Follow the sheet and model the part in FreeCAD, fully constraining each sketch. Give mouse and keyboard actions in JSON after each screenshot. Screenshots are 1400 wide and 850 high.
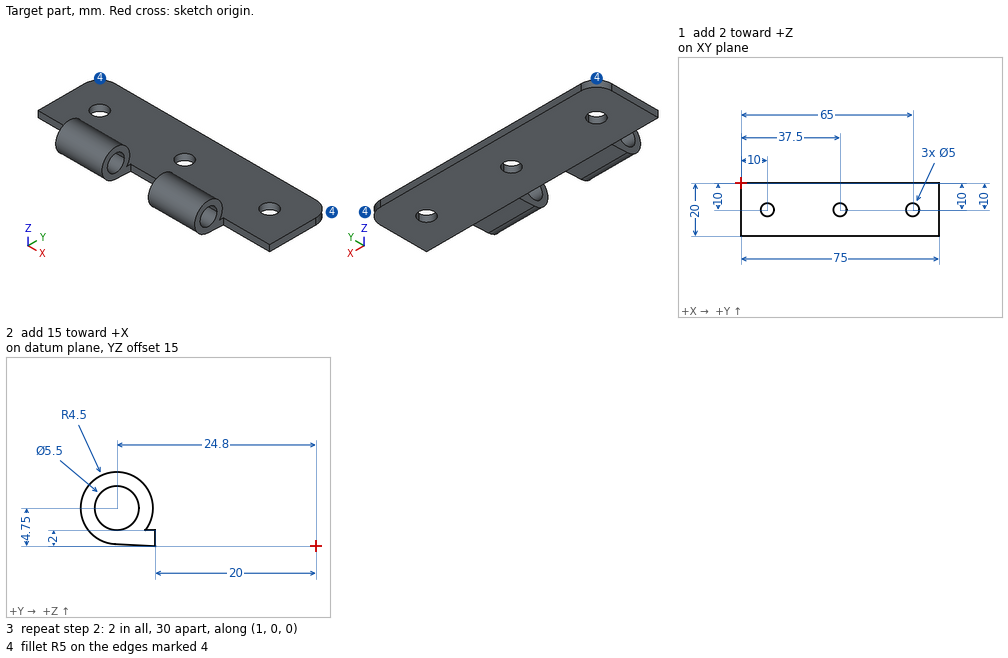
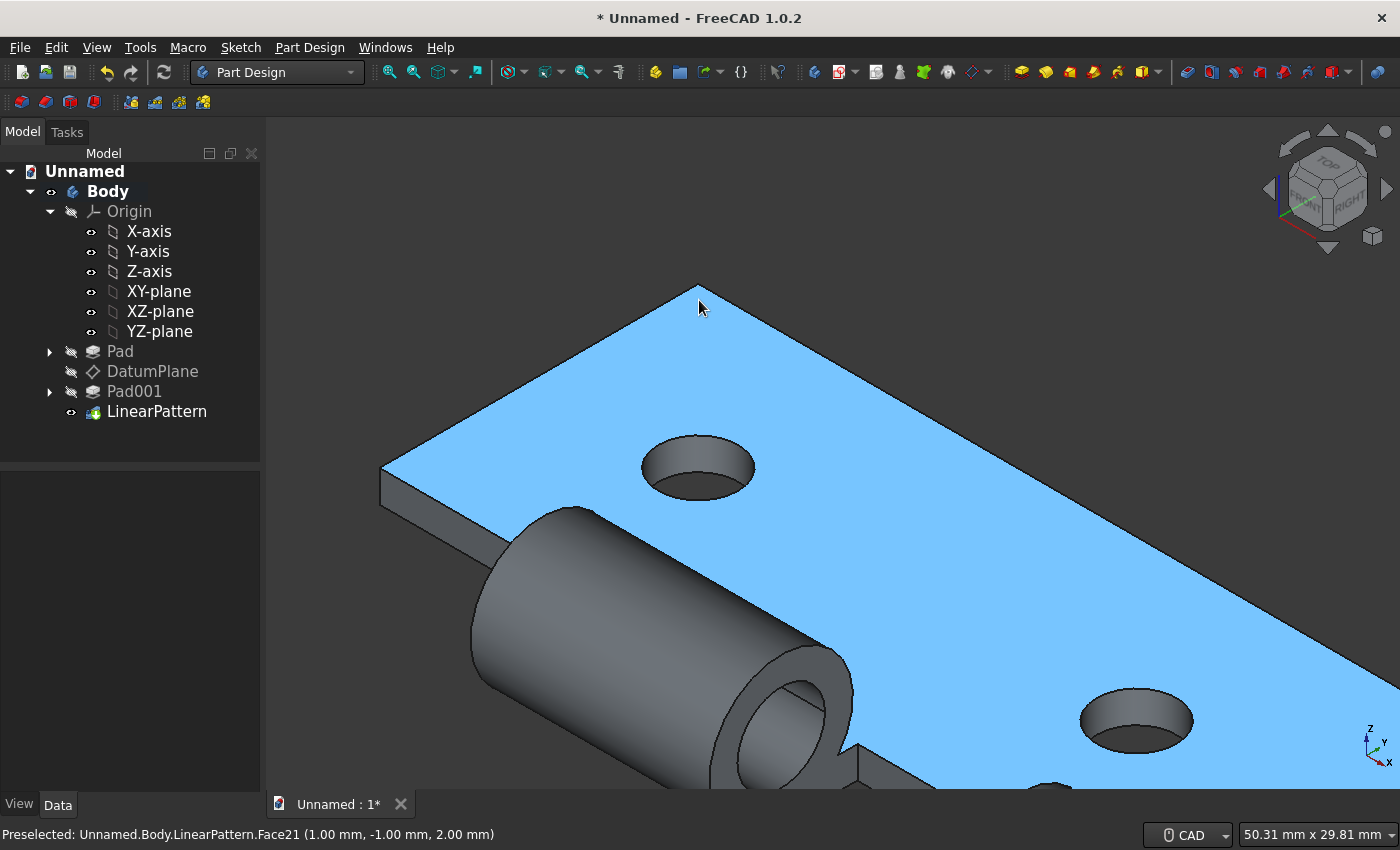
{"action": "key", "text": "v f"}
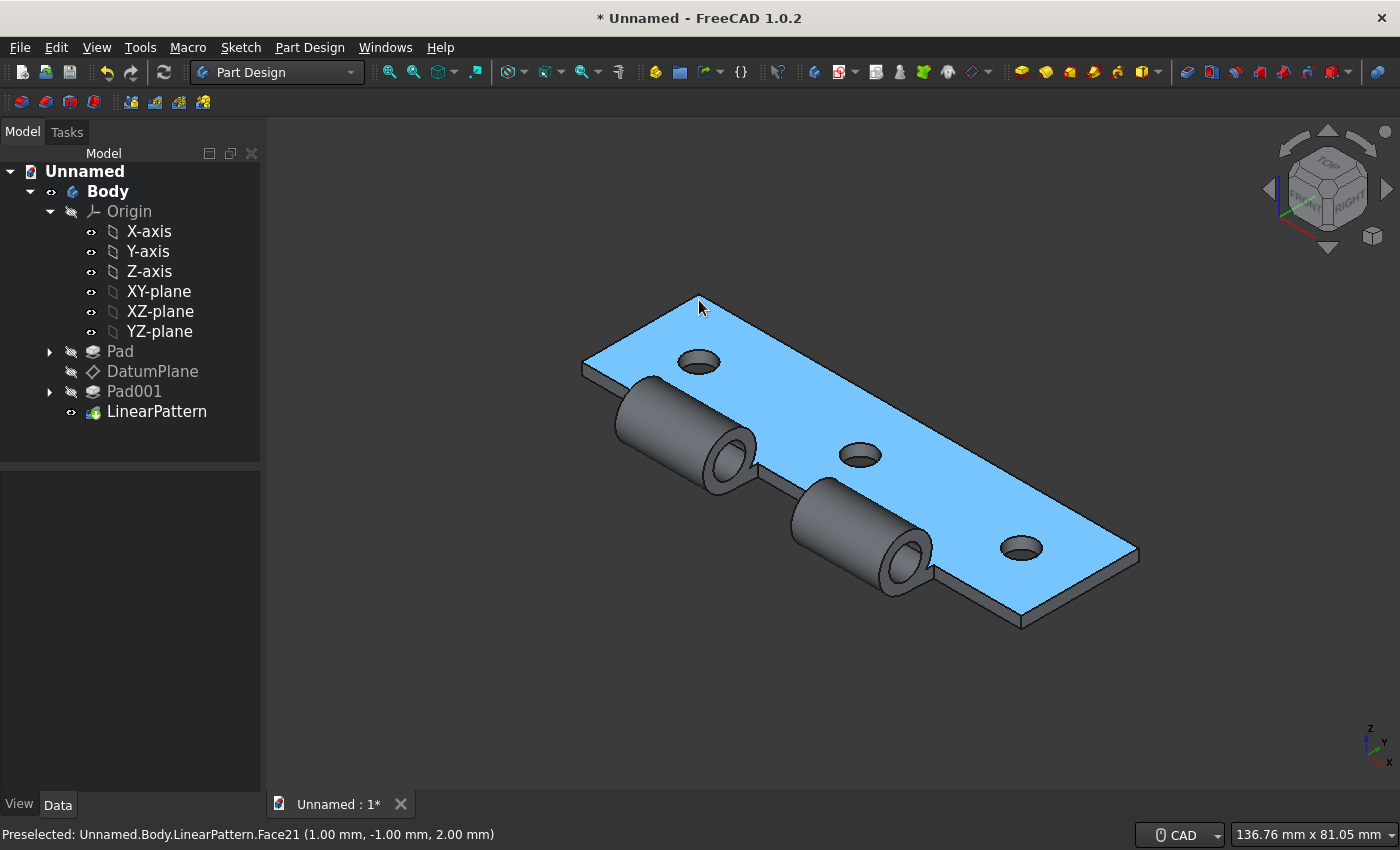
{"action": "key", "text": "2"}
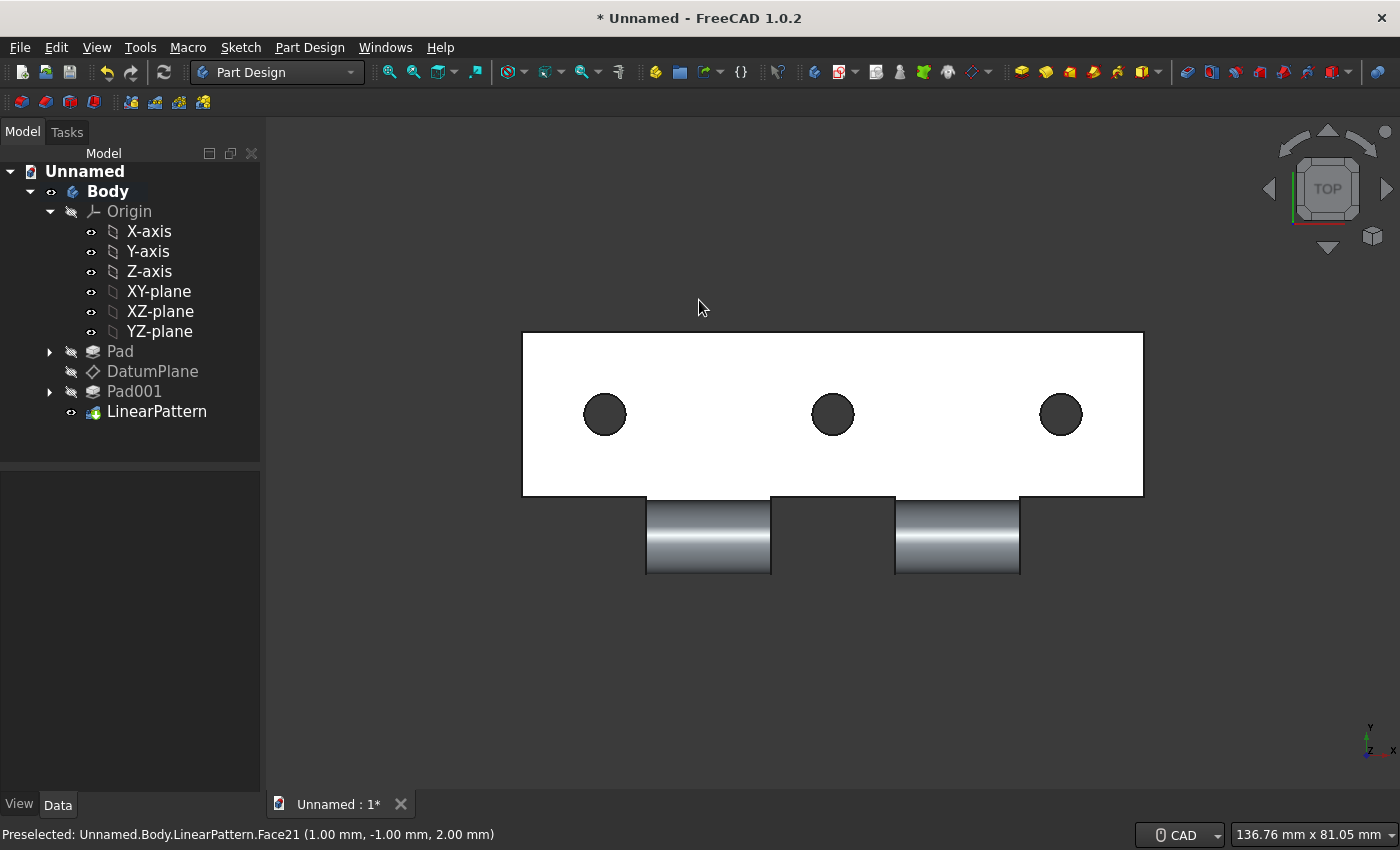
{"action": "scroll", "coordinate": [522, 331], "scroll_direction": "up", "scroll_amount": 5}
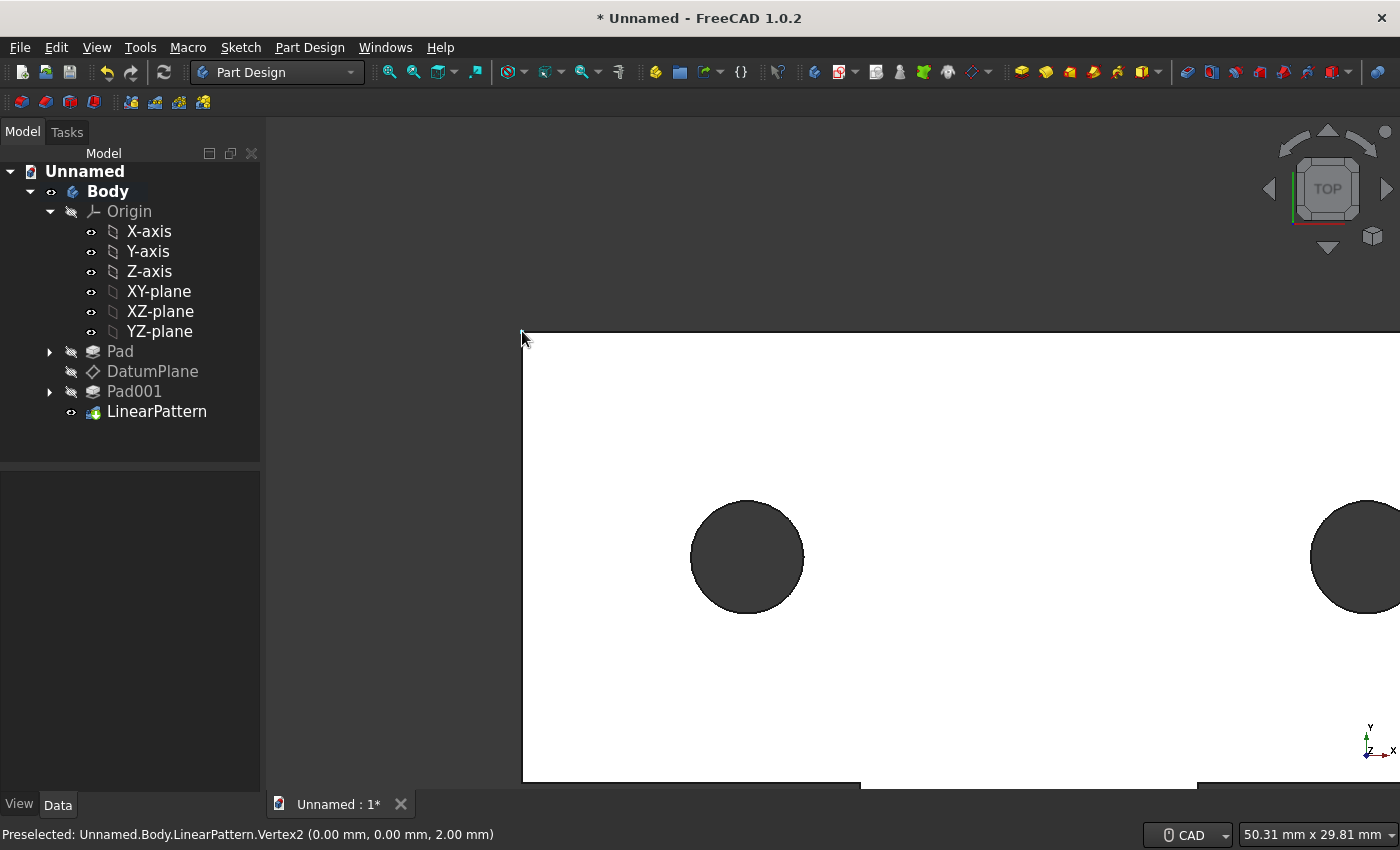
{"action": "key", "text": "v f"}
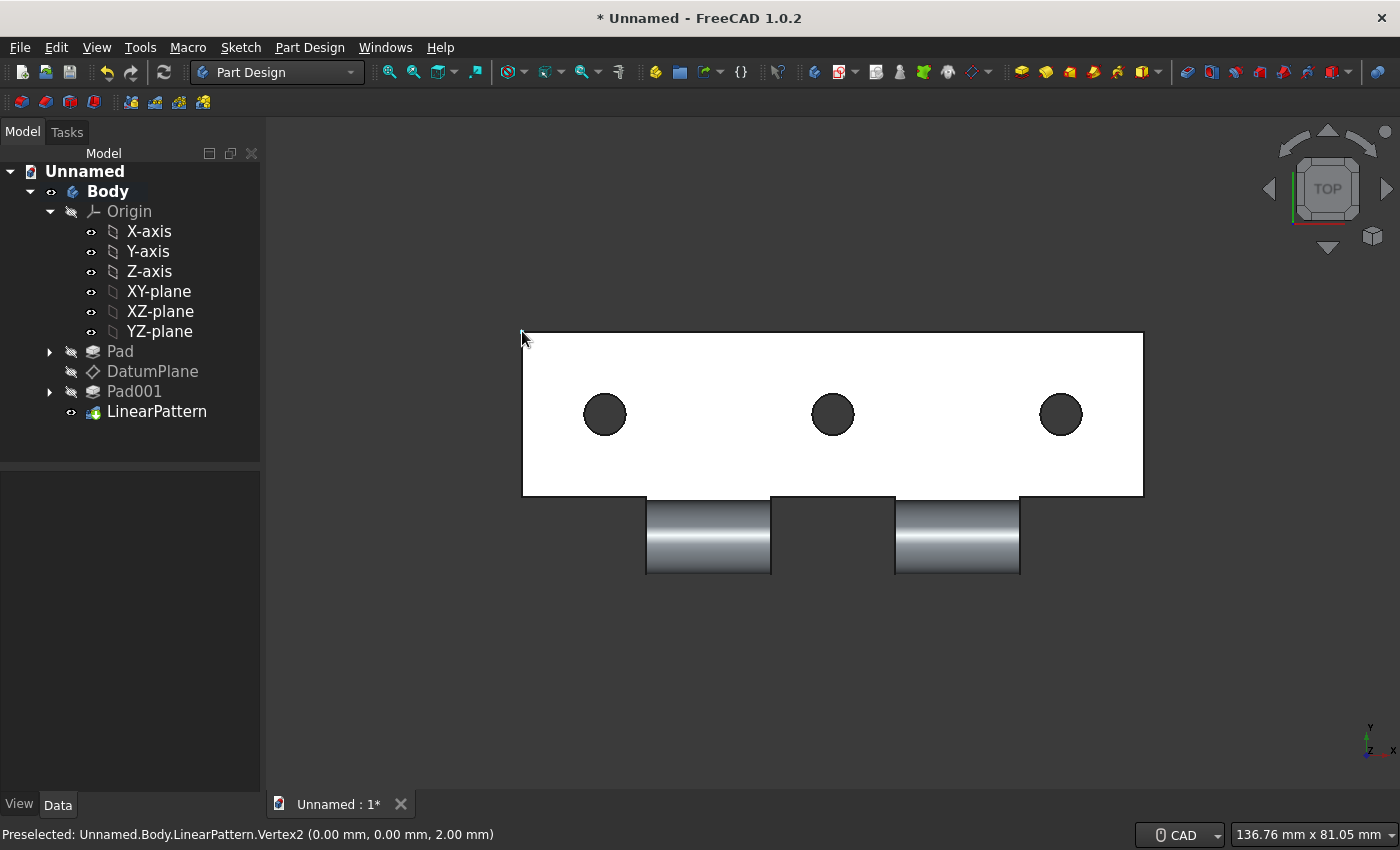
{"action": "key", "text": "1"}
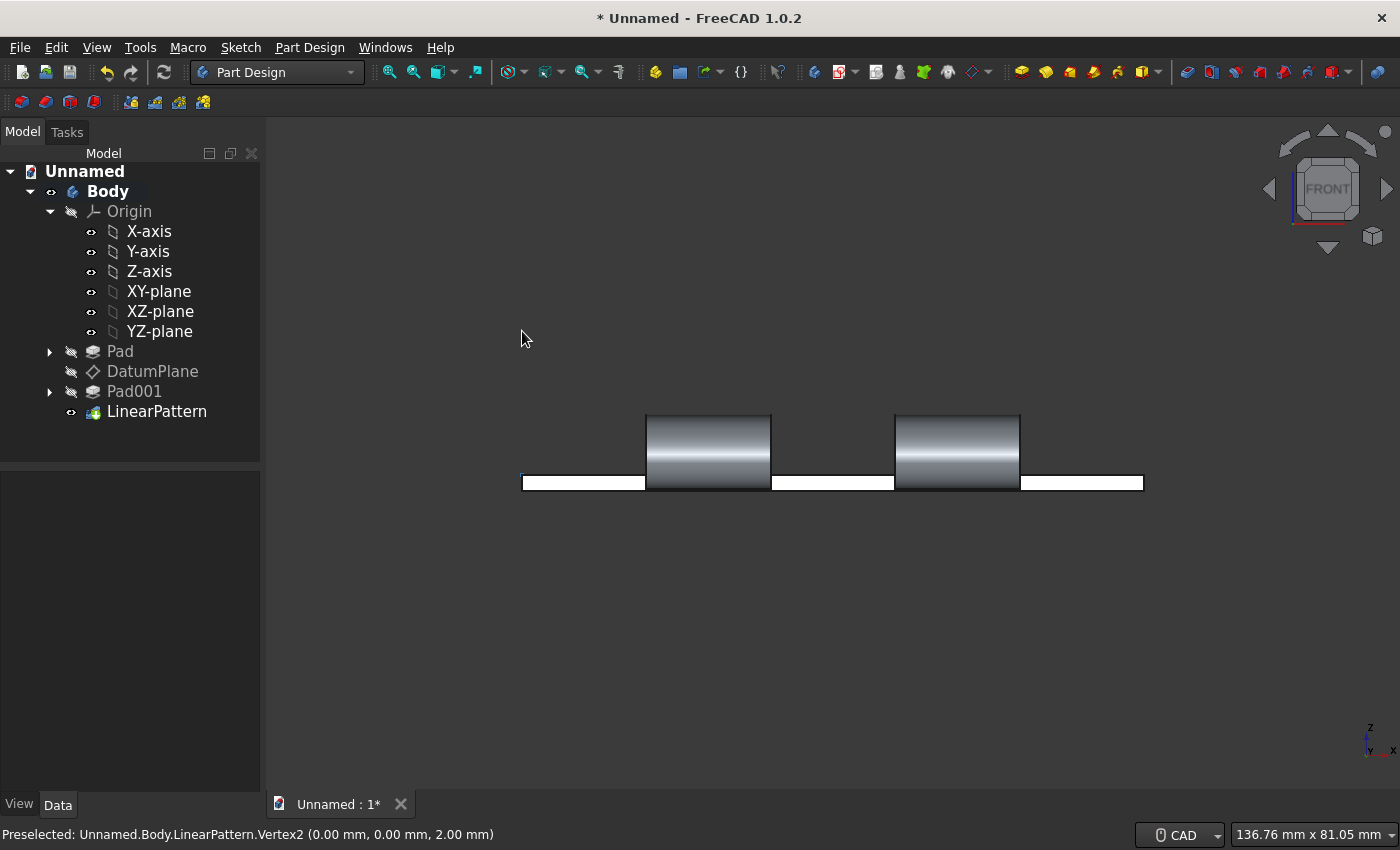
{"action": "scroll", "coordinate": [522, 482], "scroll_direction": "up", "scroll_amount": 5}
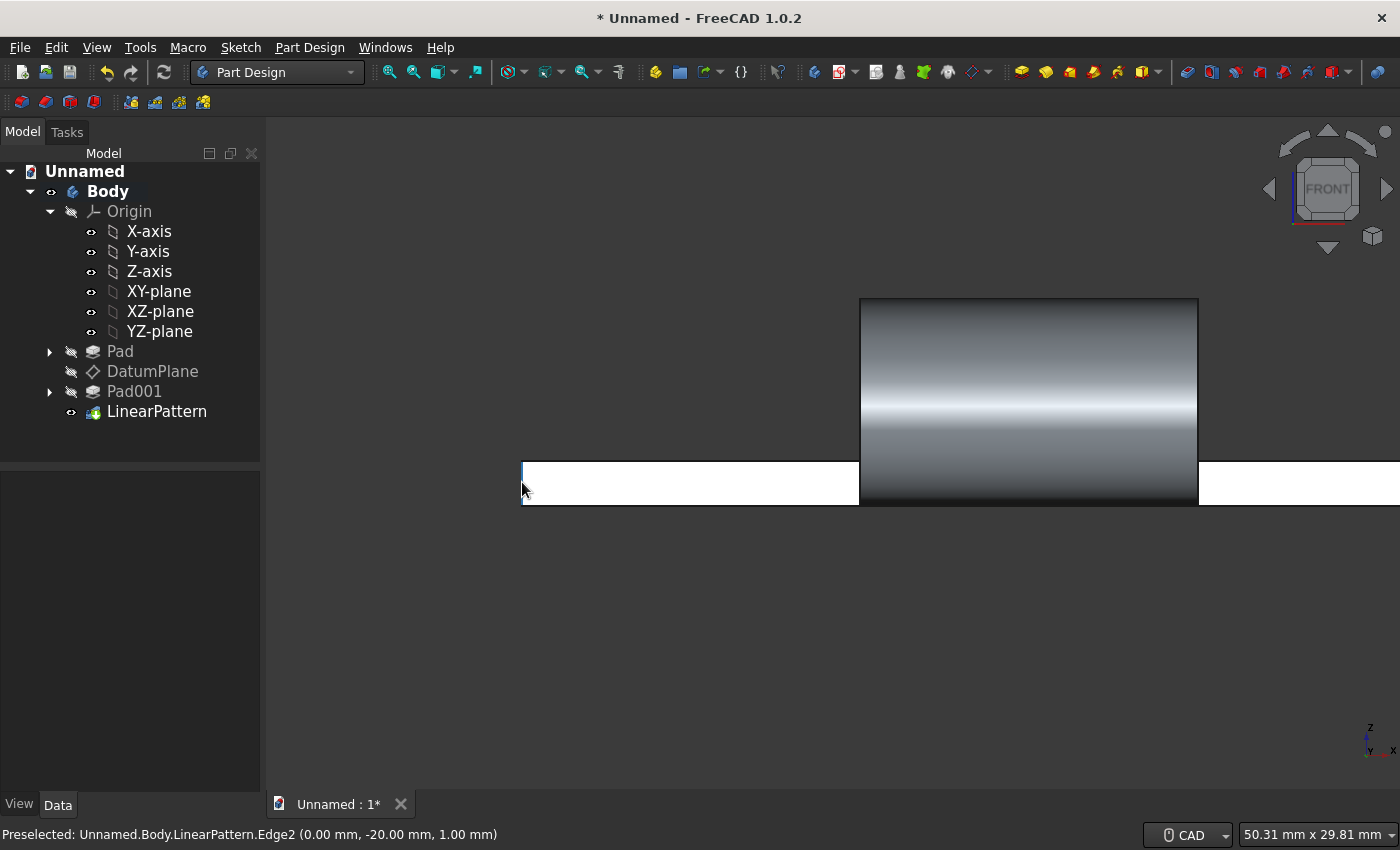
{"action": "key", "text": "v f"}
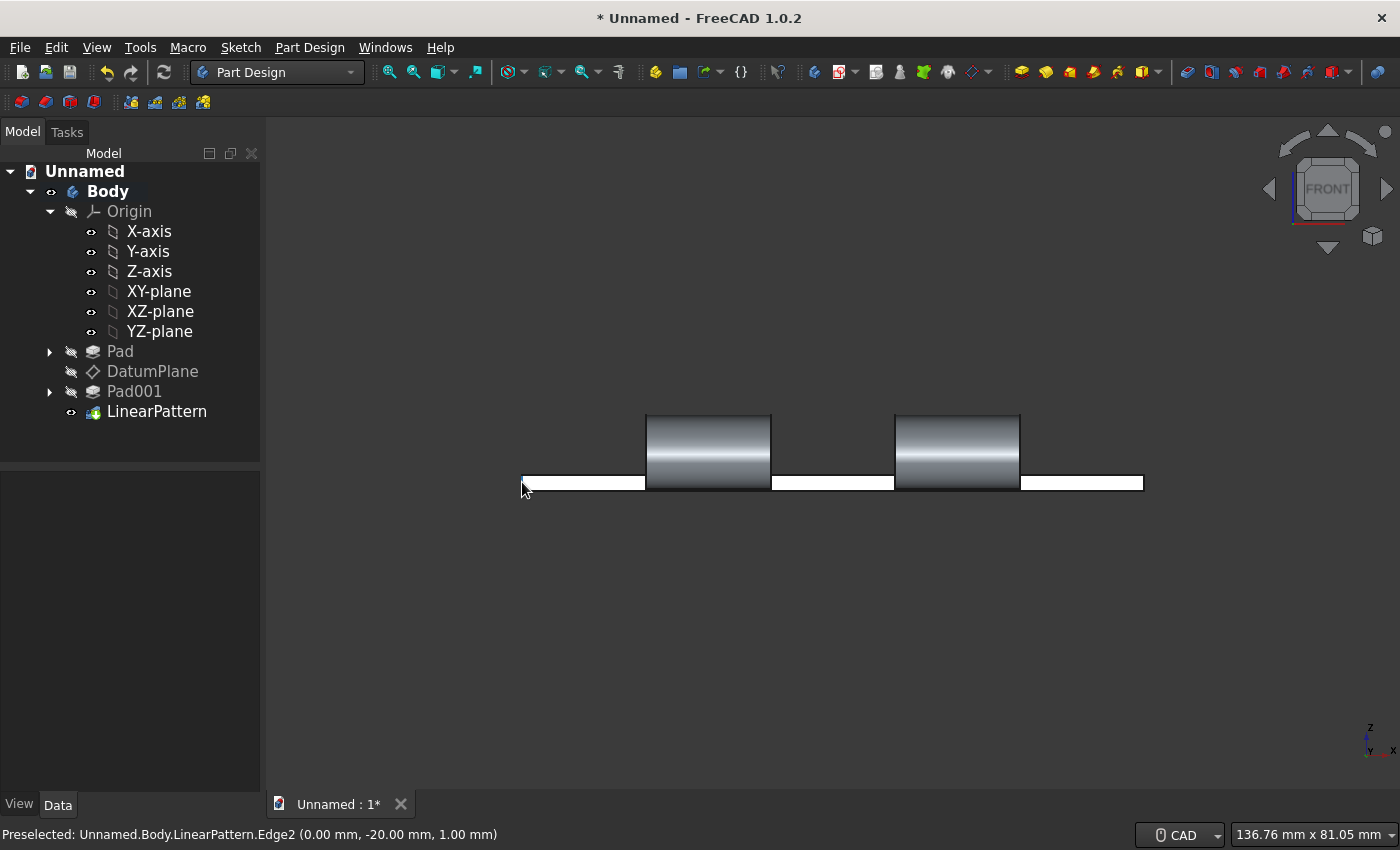
{"action": "key", "text": "3"}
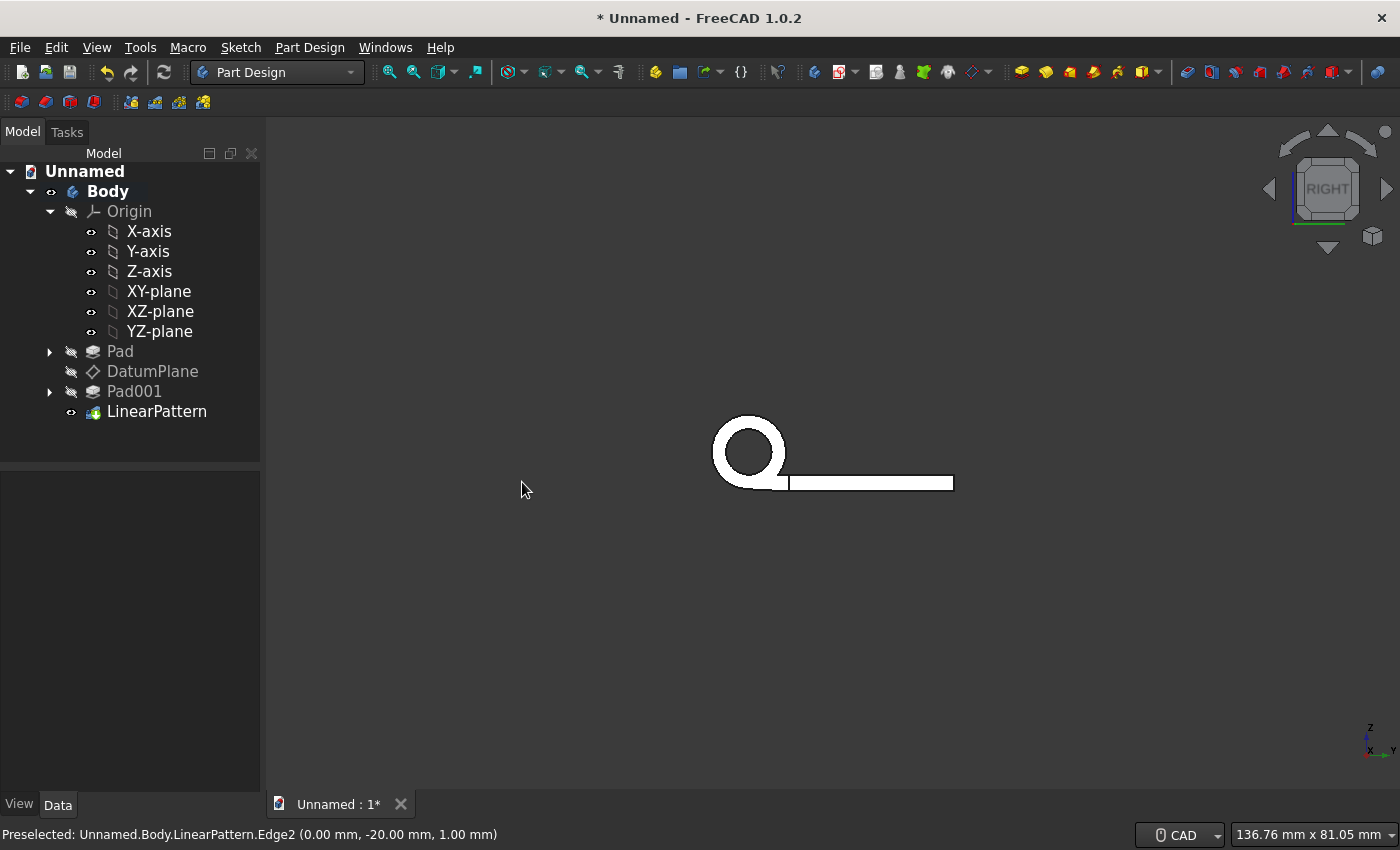
{"action": "key", "text": "v f"}